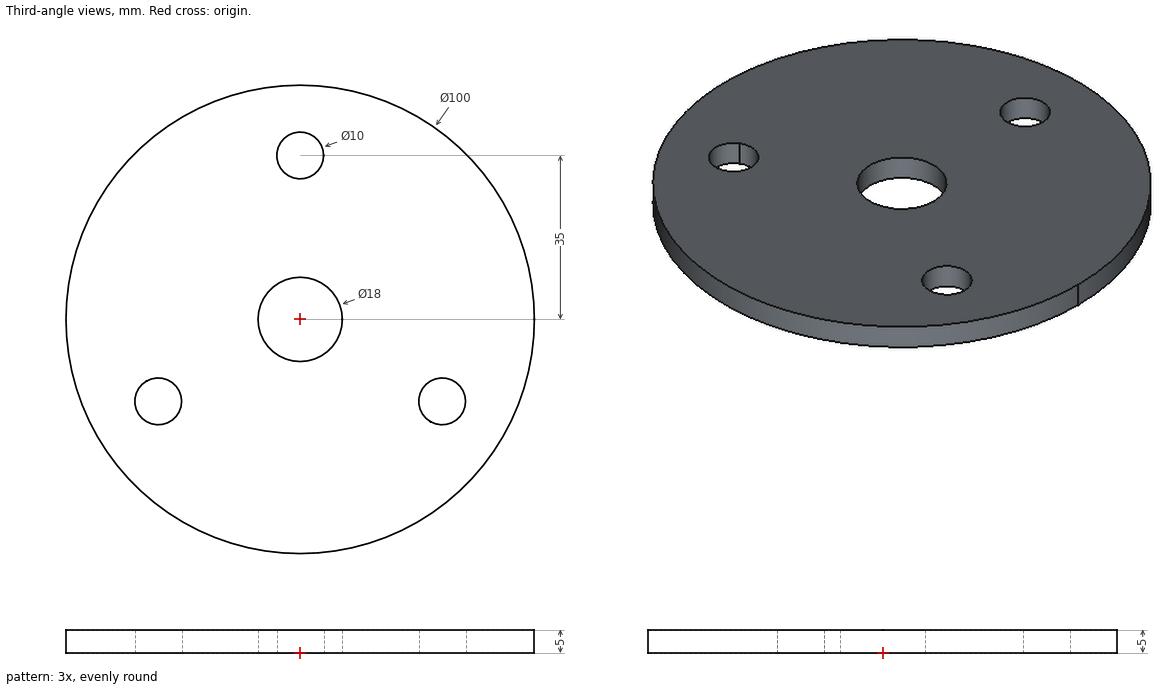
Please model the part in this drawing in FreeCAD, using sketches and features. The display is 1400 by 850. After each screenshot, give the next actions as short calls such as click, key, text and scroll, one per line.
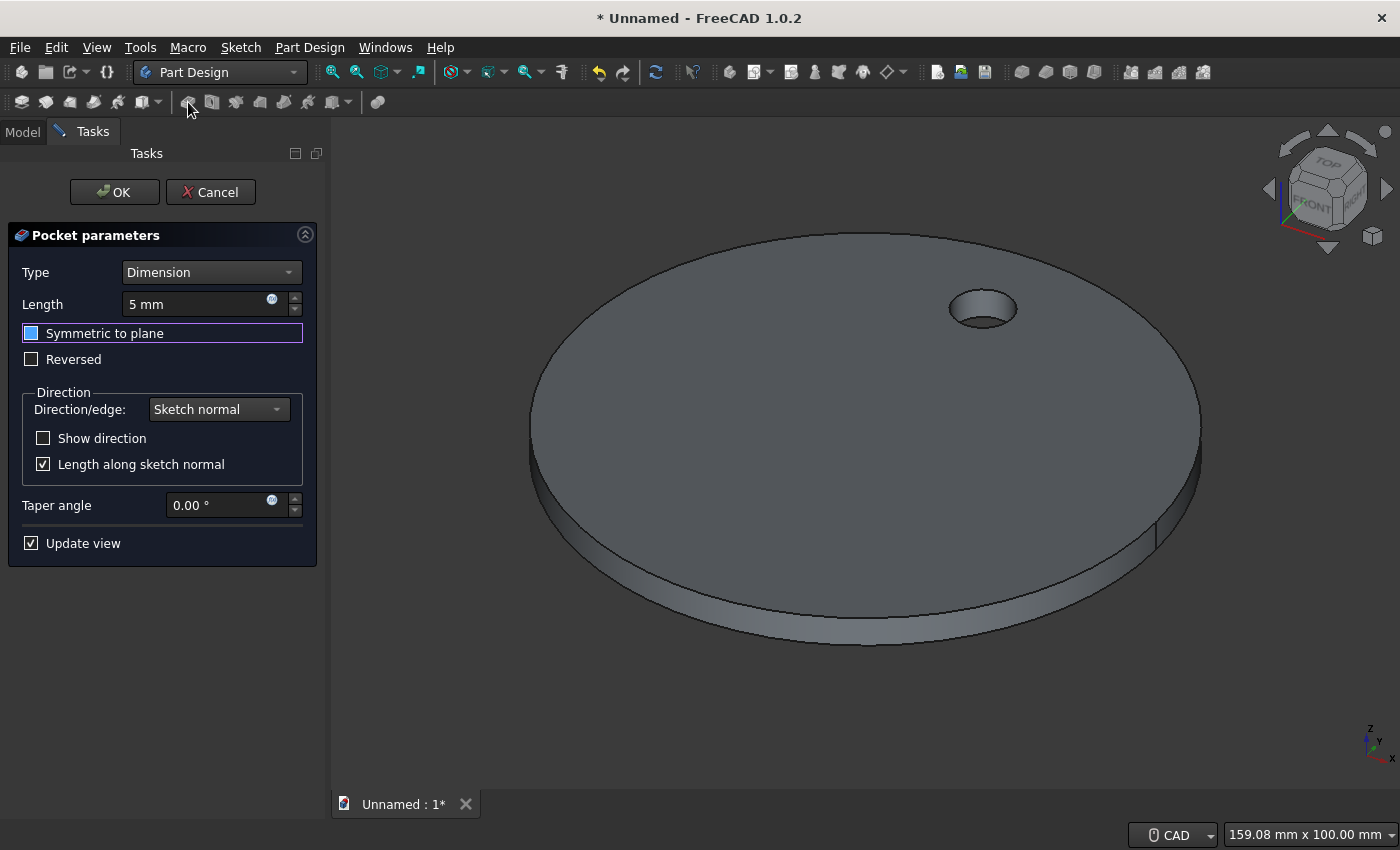
click(115, 192)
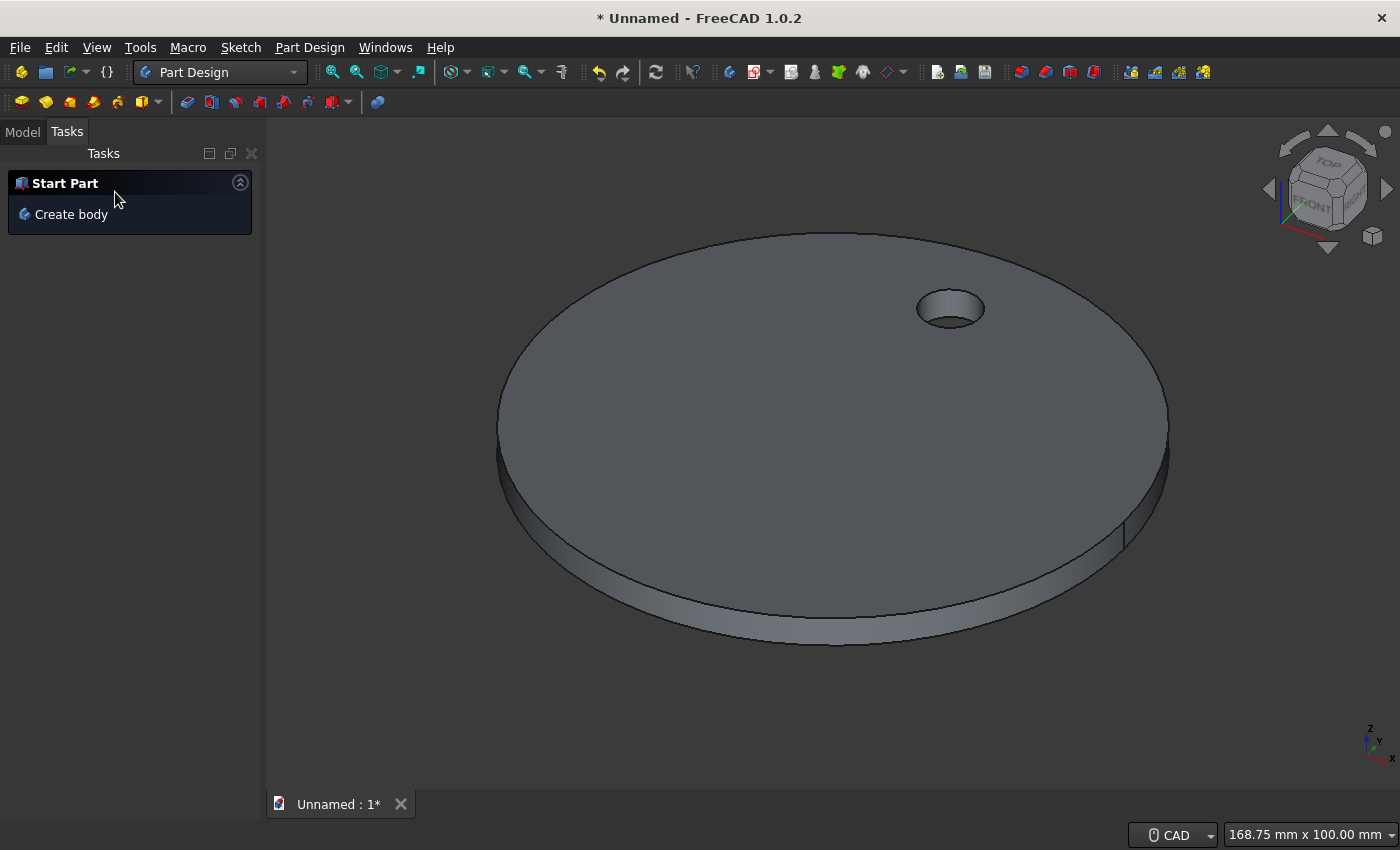
click(23, 131)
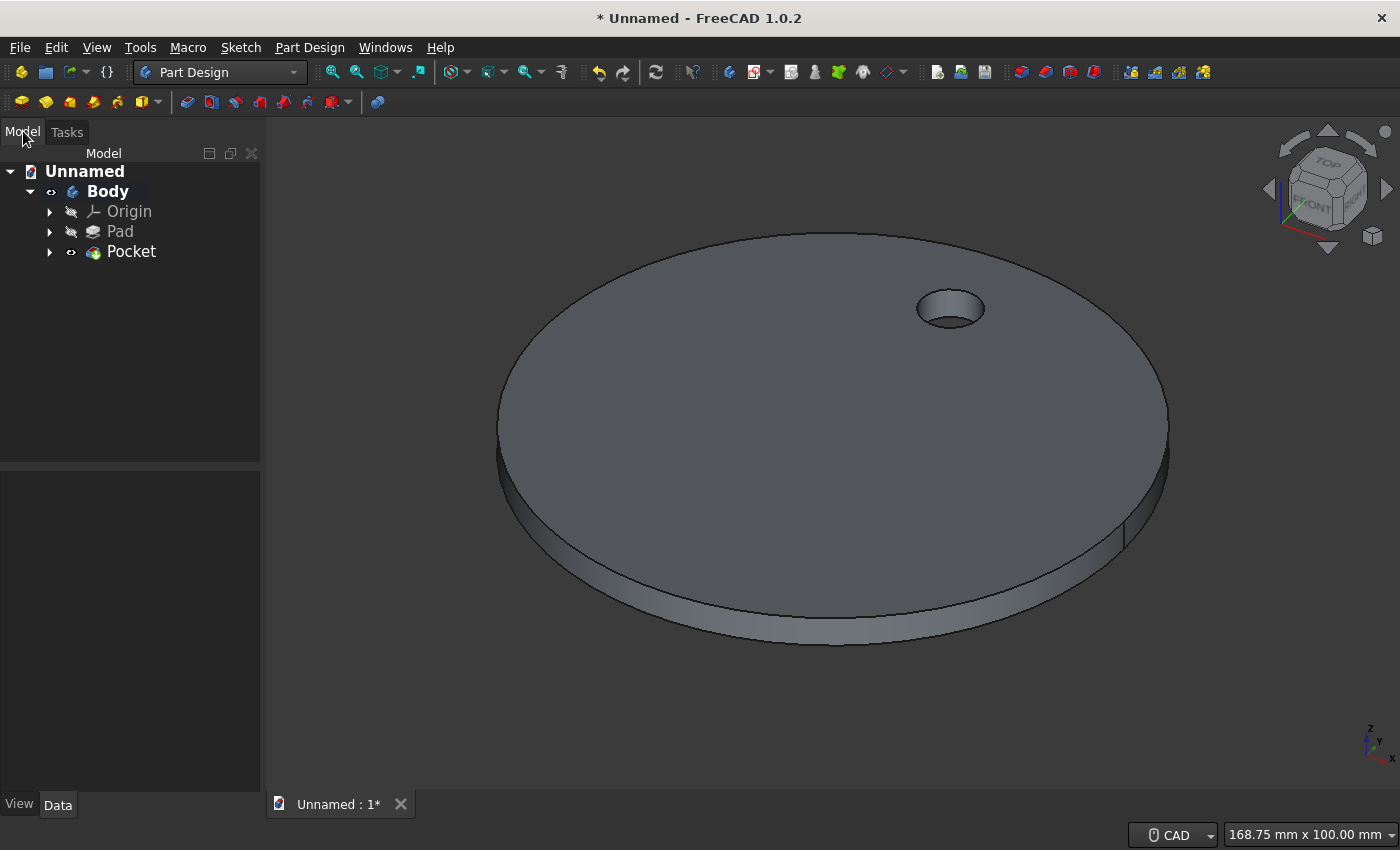
click(116, 252)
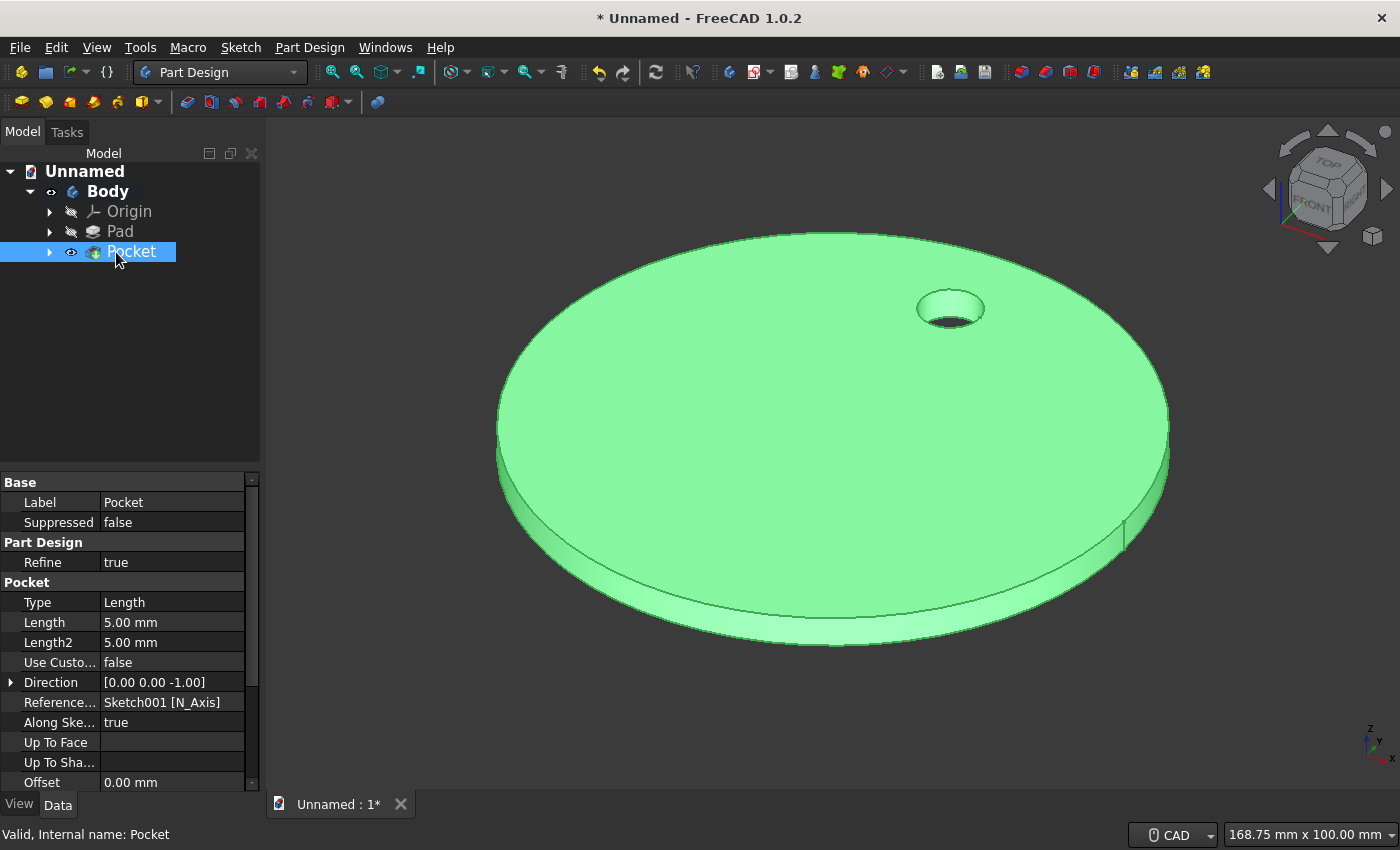
click(1180, 72)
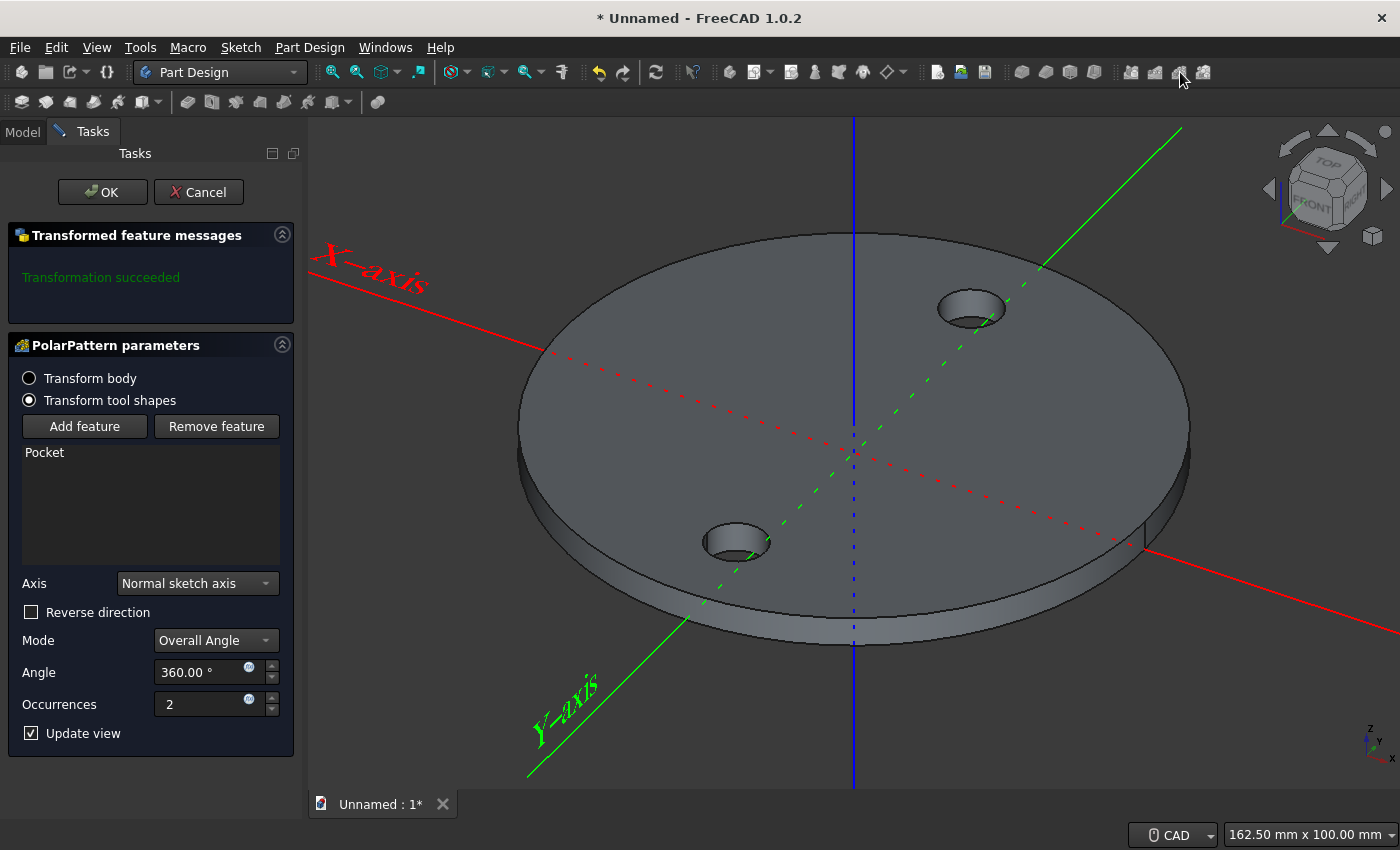
click(198, 584)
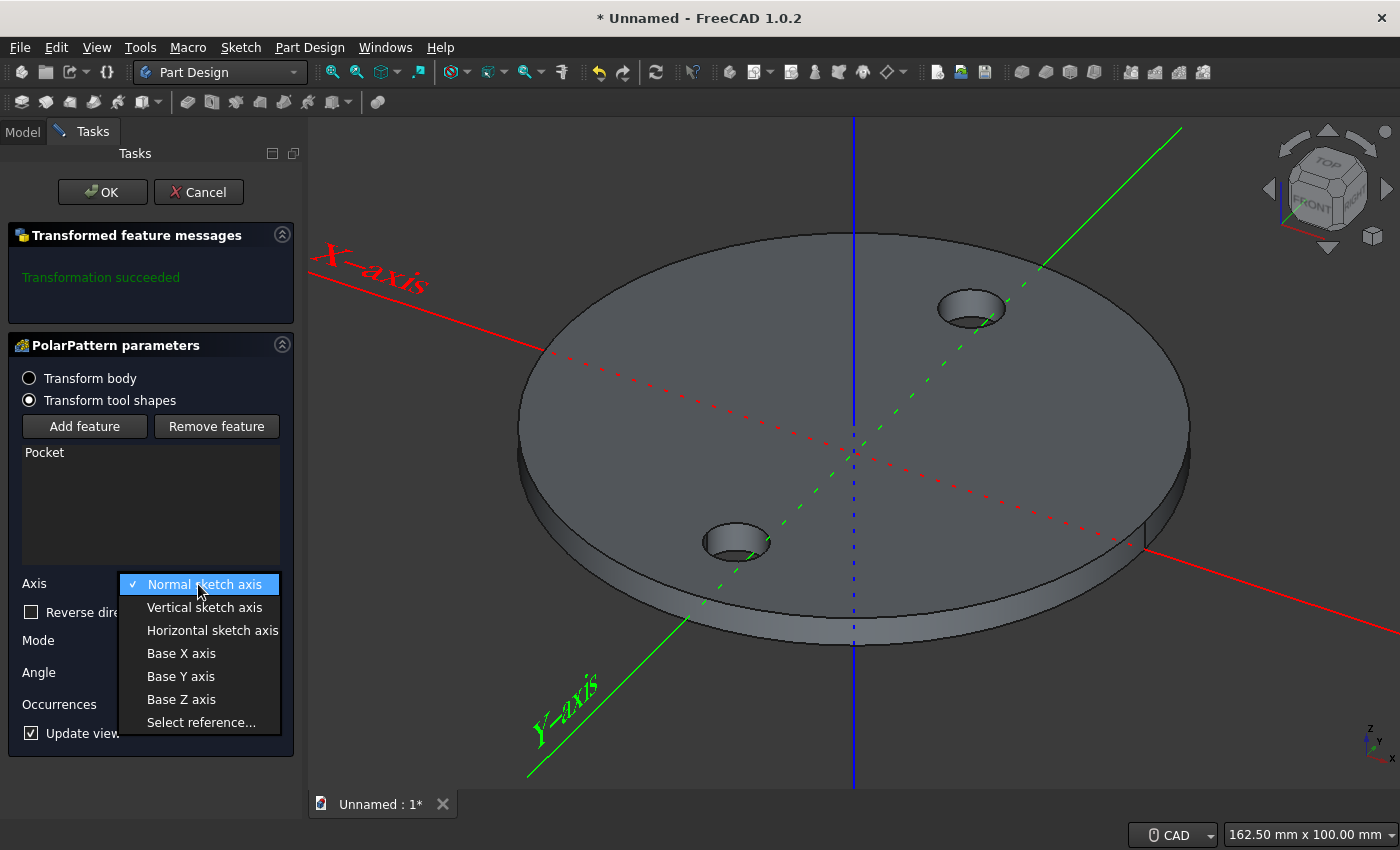
click(198, 700)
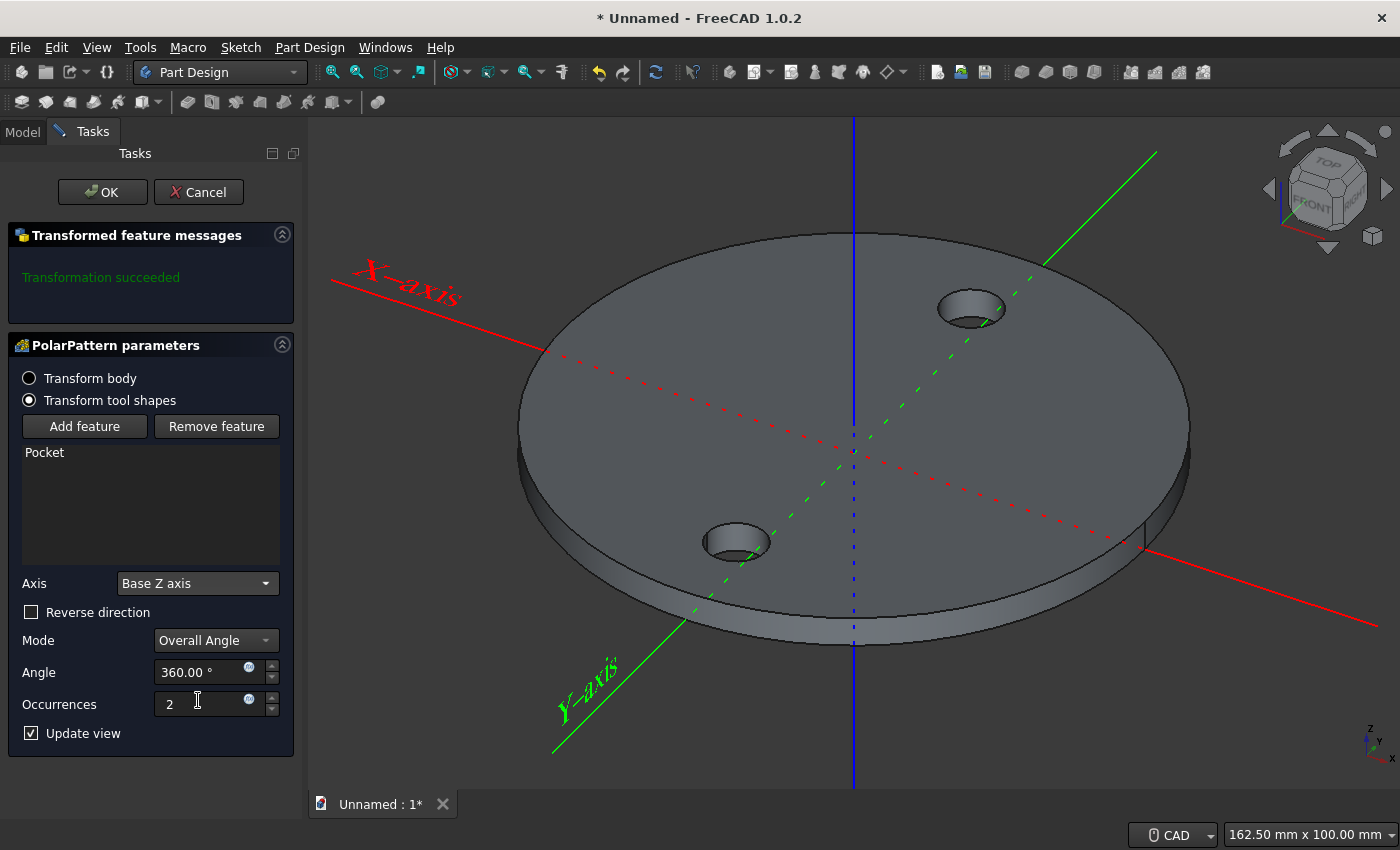
triple_click(209, 704)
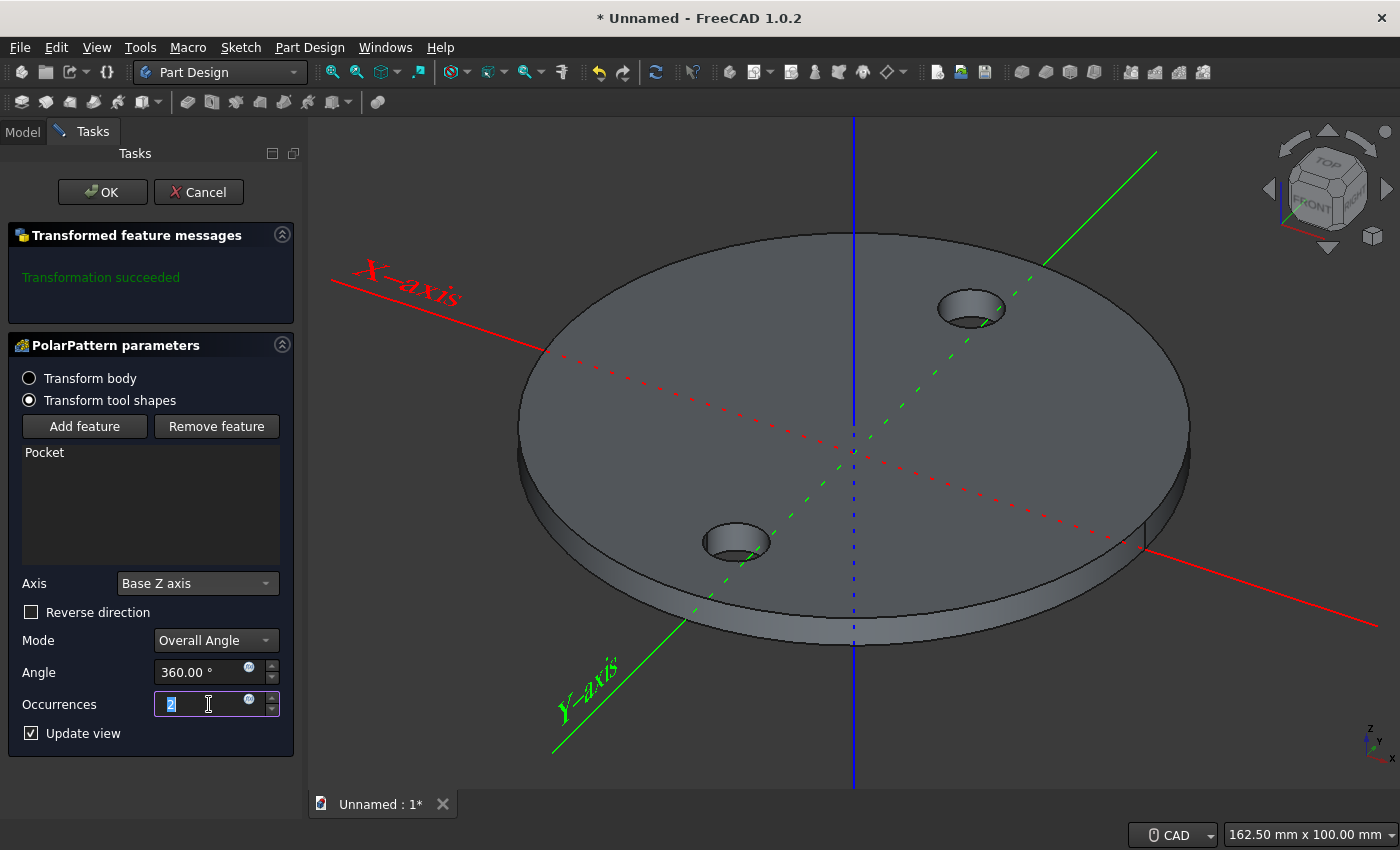
text(3)
key(Tab)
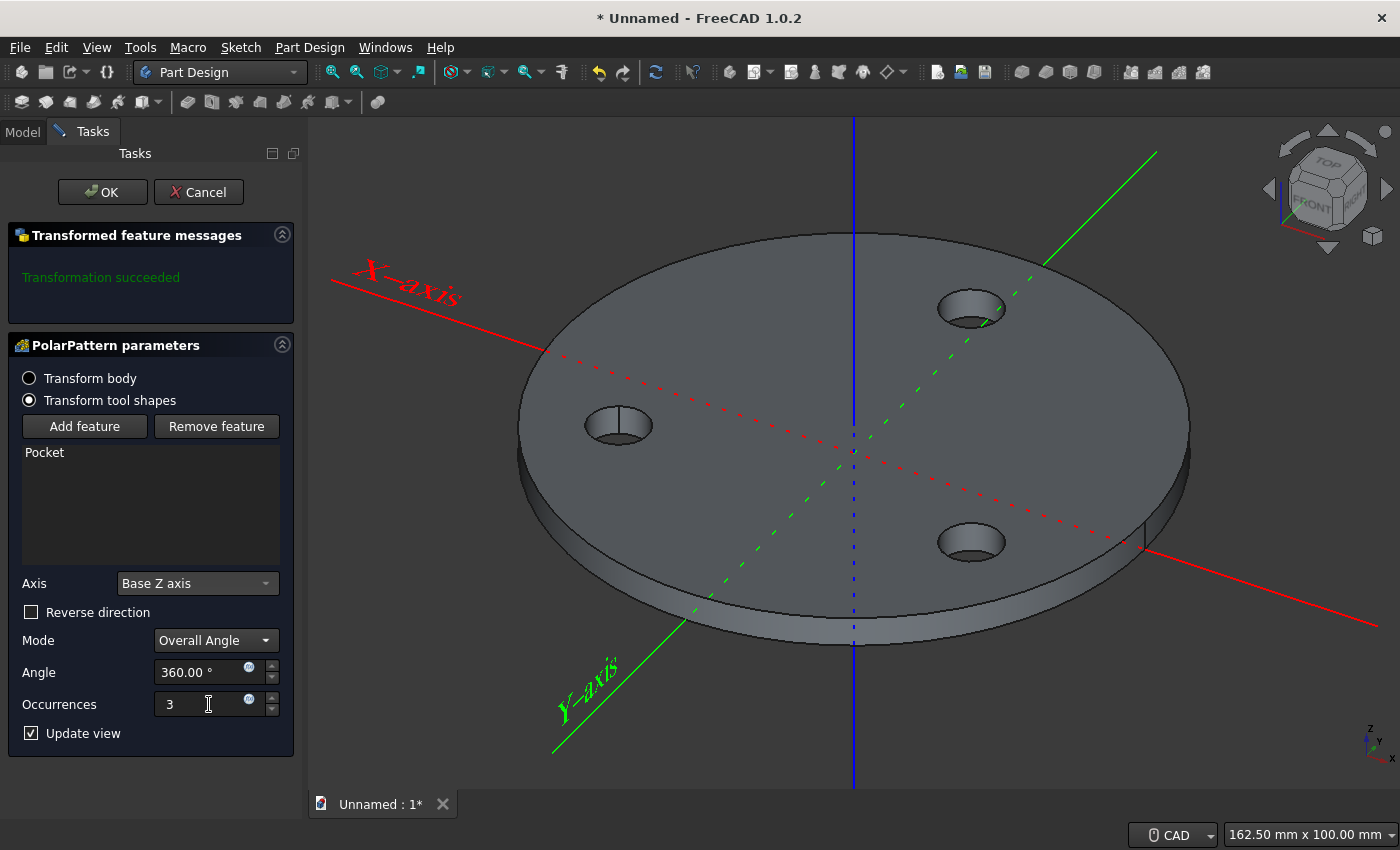
click(103, 192)